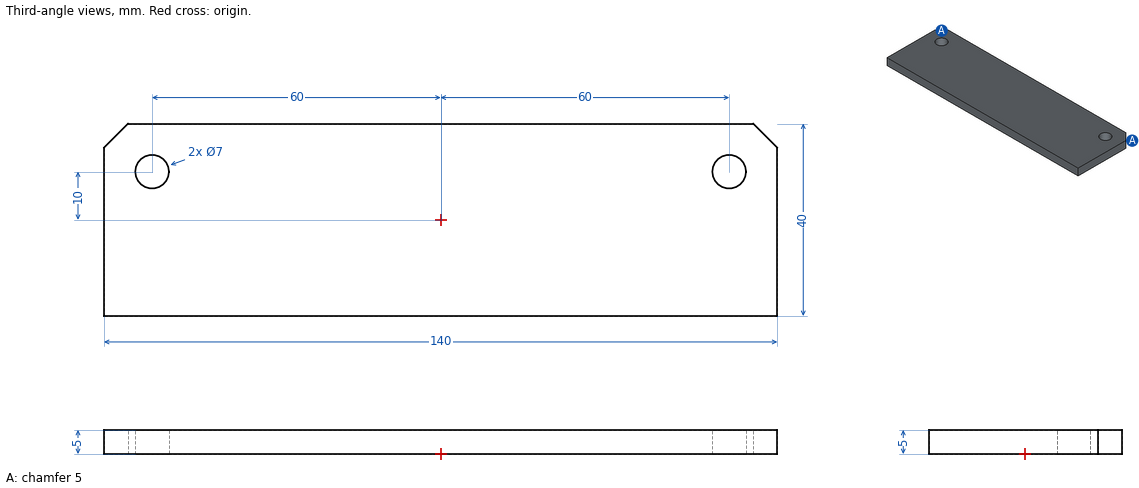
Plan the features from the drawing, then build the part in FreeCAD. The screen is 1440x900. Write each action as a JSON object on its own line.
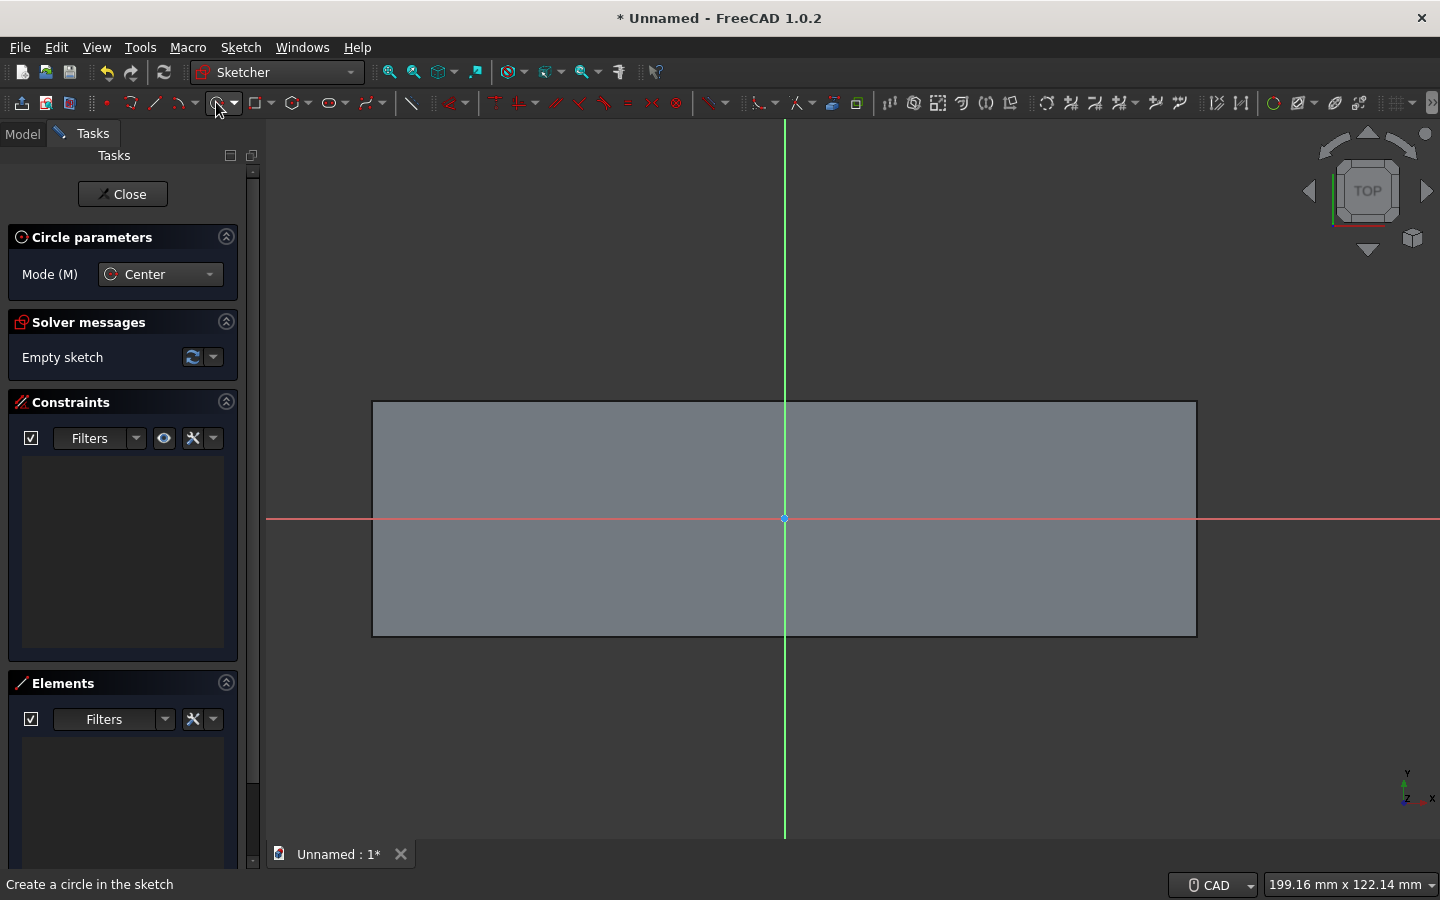
{"action": "left_click", "coordinate": [431, 460]}
{"action": "mouse_move", "coordinate": [446, 445]}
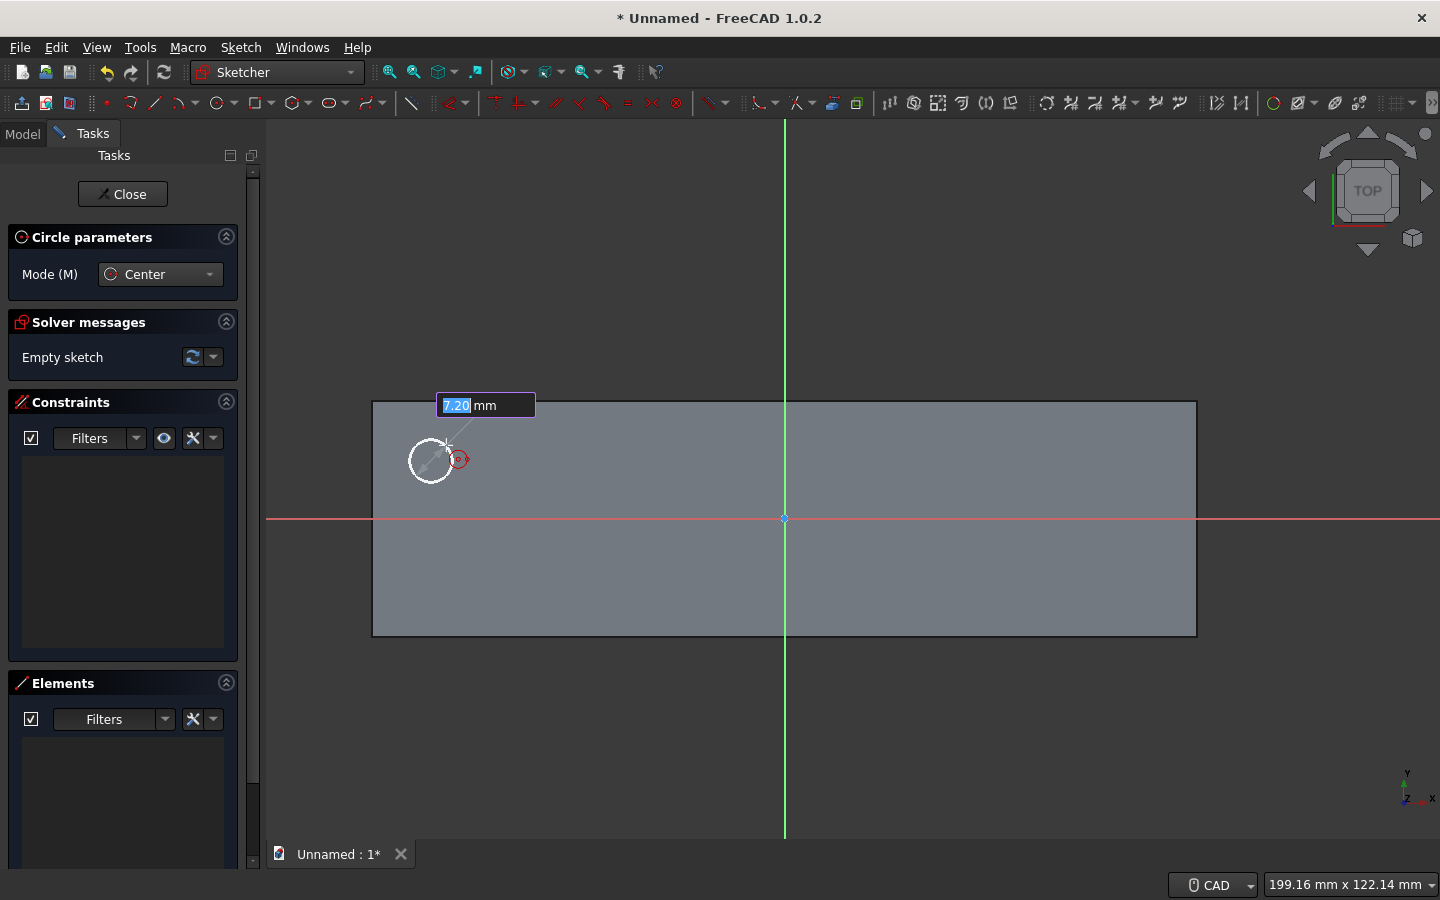
{"action": "type", "text": "7"}
{"action": "key", "text": "Return"}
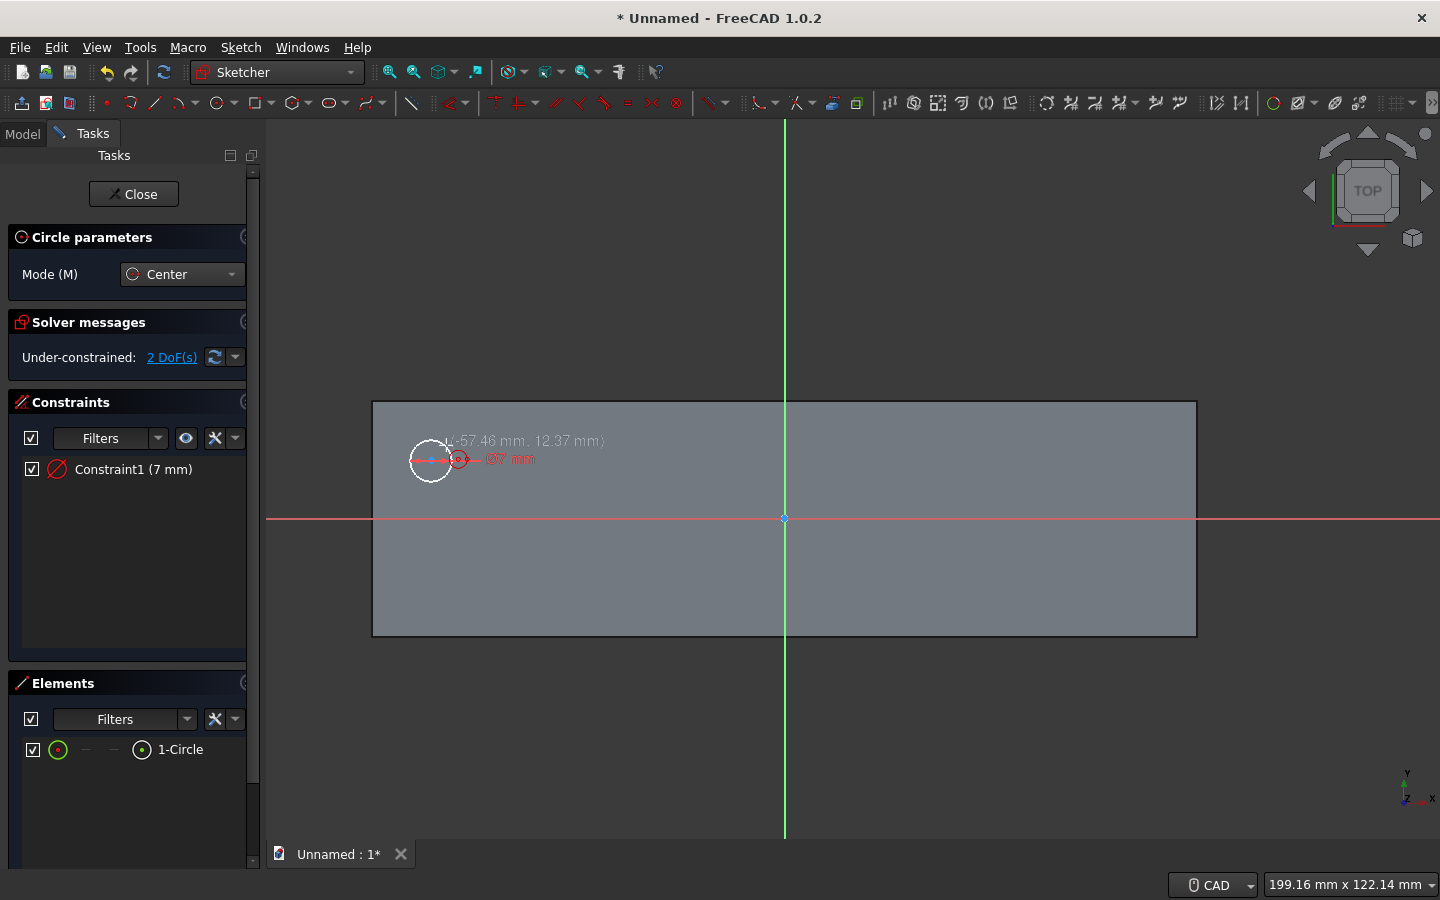
{"action": "left_click", "coordinate": [1138, 460]}
{"action": "mouse_move", "coordinate": [1153, 445]}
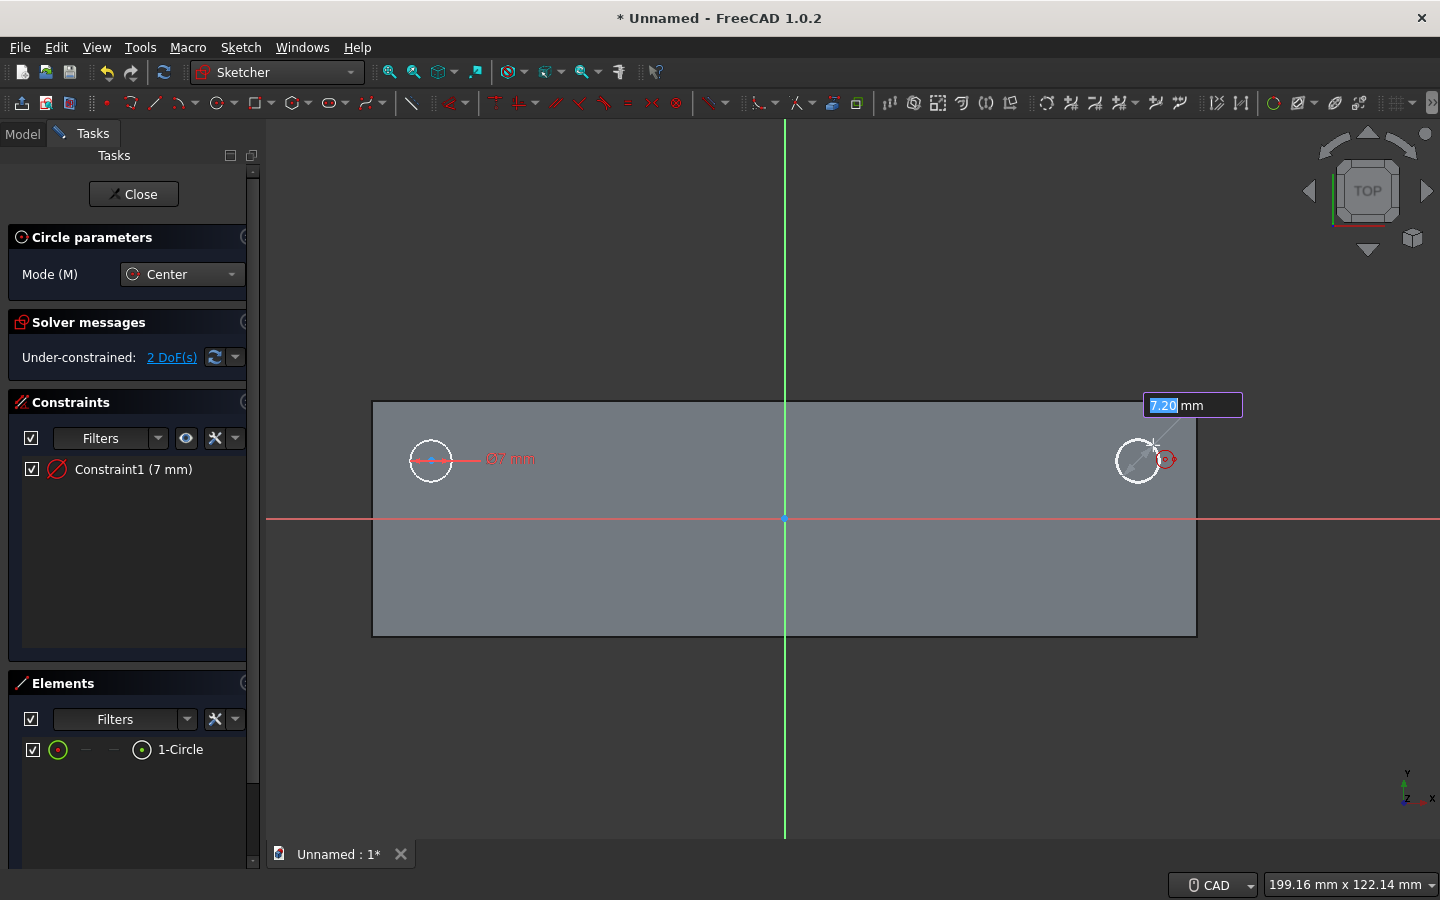
{"action": "type", "text": "7"}
{"action": "key", "text": "Return"}
{"action": "key", "text": "Escape"}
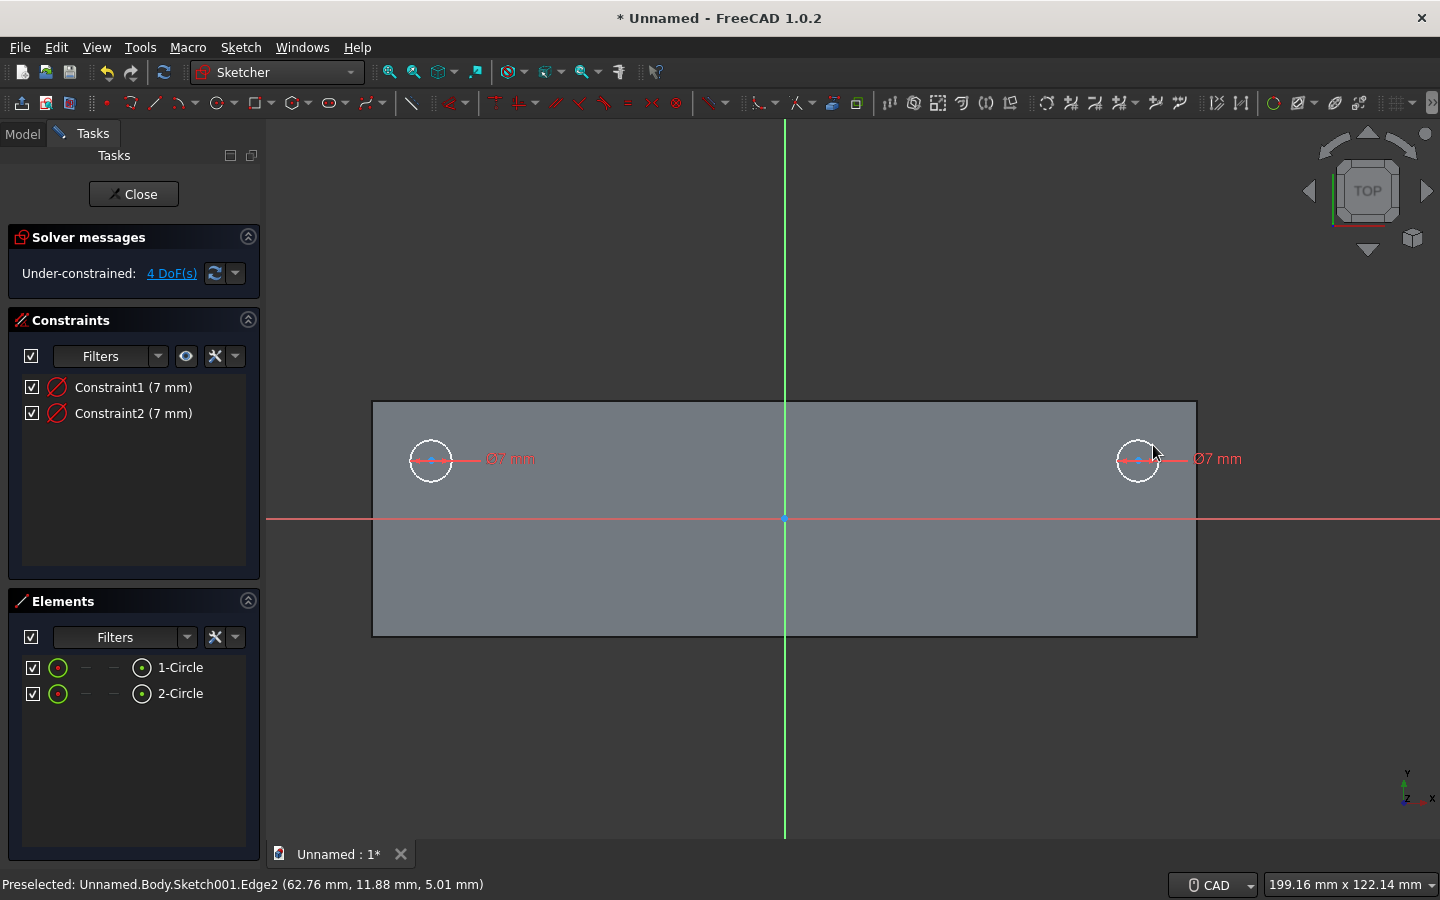
{"action": "left_click", "coordinate": [431, 461]}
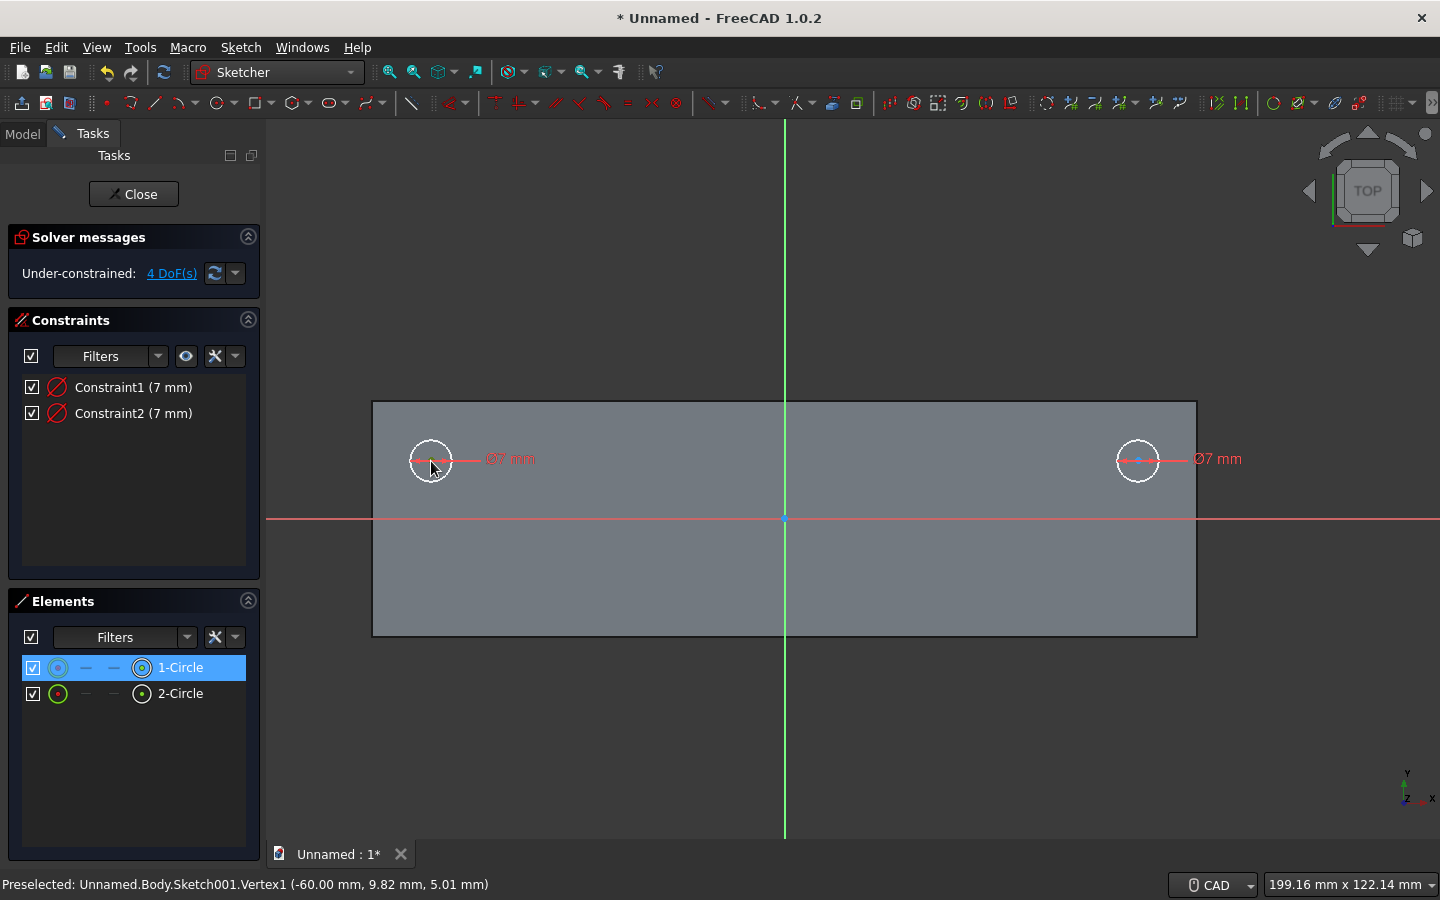
{"action": "left_click", "coordinate": [1138, 461]}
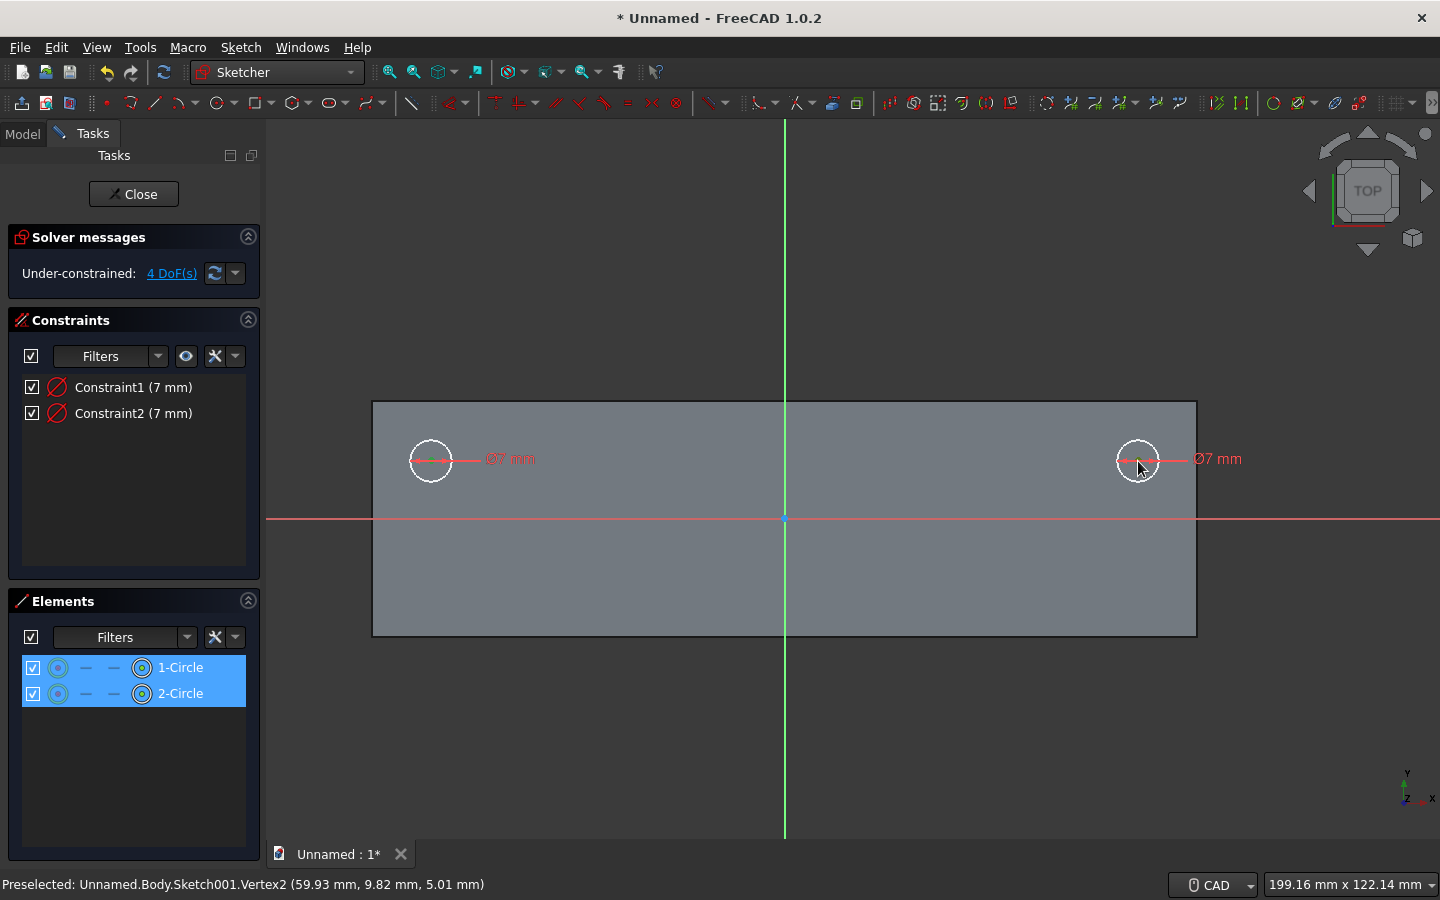
{"action": "key", "text": "h"}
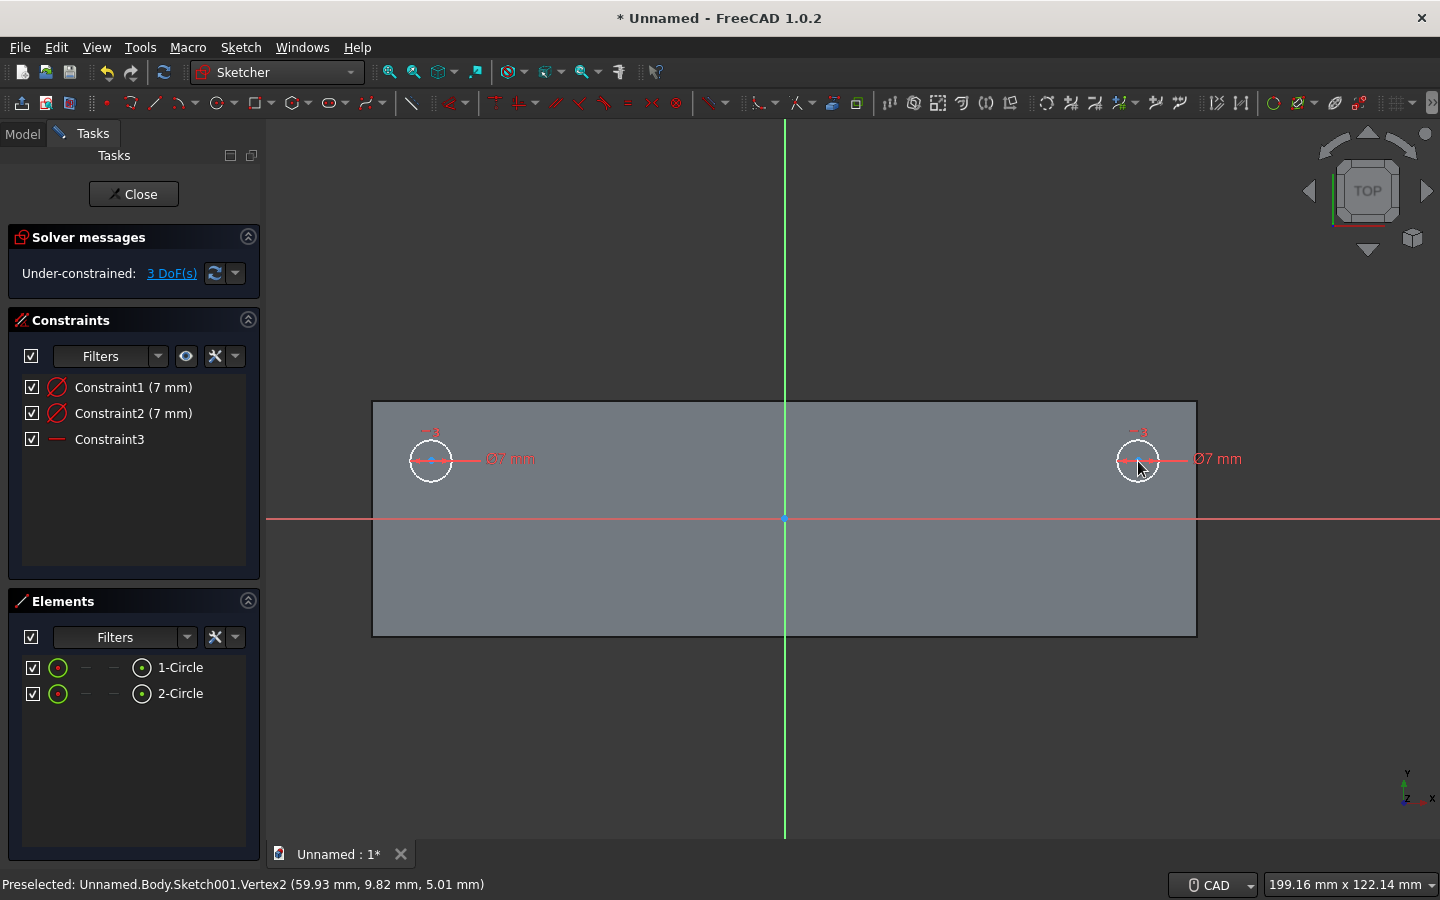
{"action": "left_click", "coordinate": [450, 104]}